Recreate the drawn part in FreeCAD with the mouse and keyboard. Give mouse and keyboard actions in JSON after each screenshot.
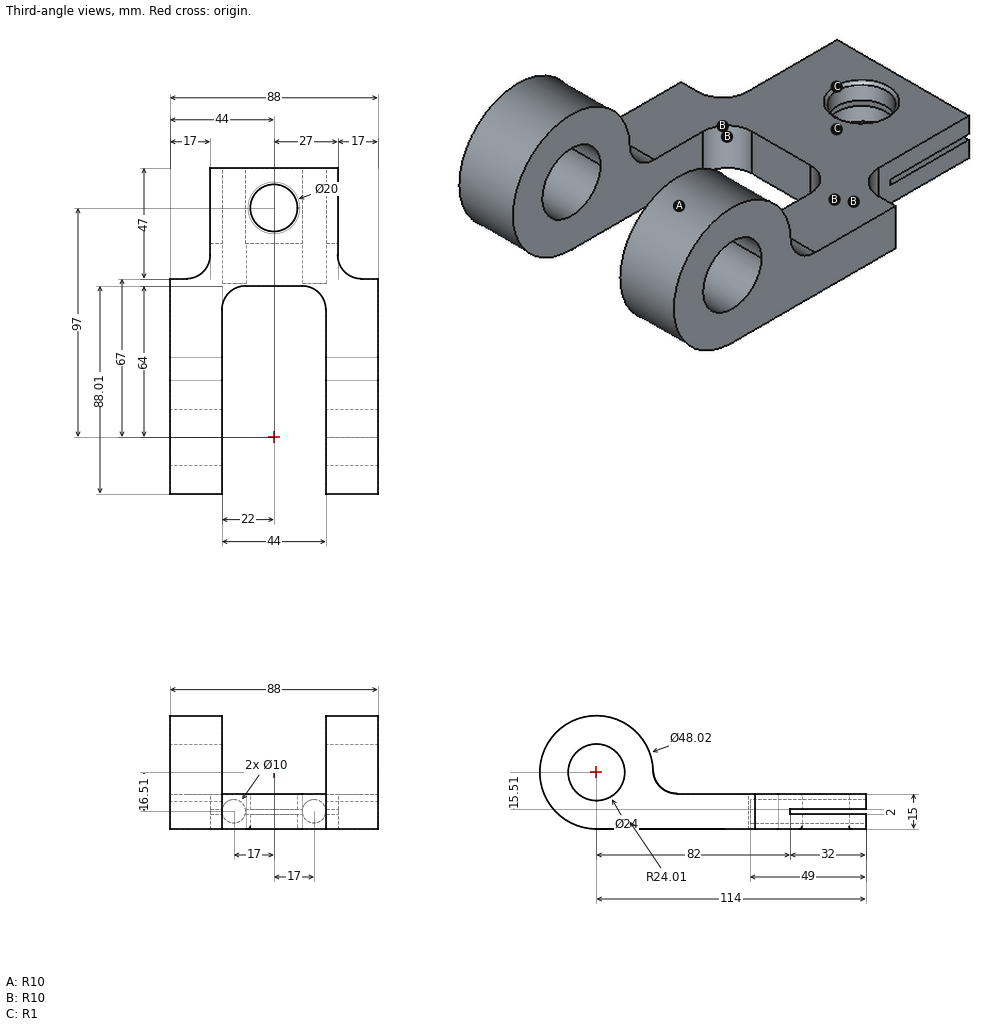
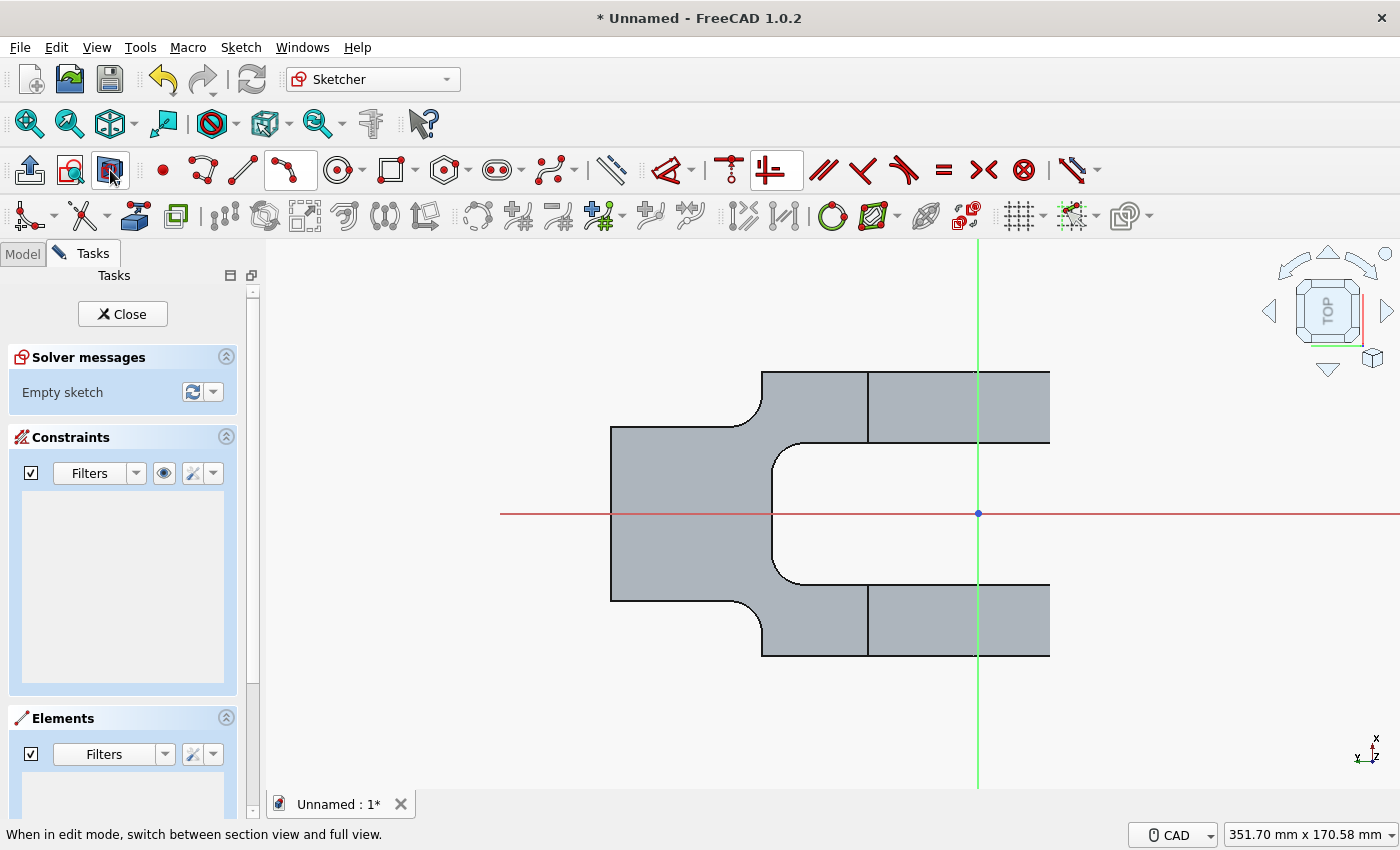
{"action": "scroll", "coordinate": [640, 514], "scroll_direction": "up", "scroll_amount": 8}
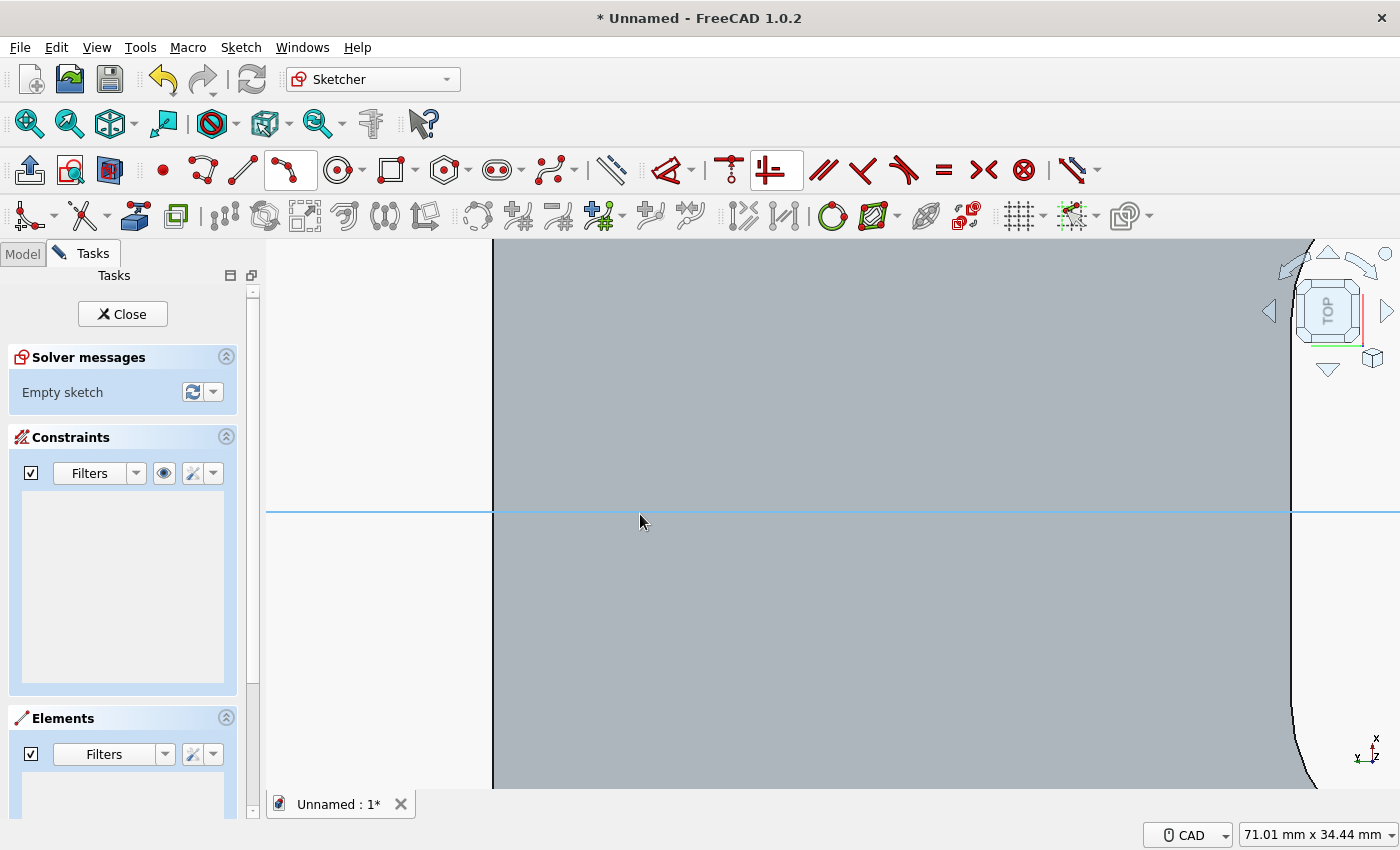
{"action": "left_click", "coordinate": [338, 170]}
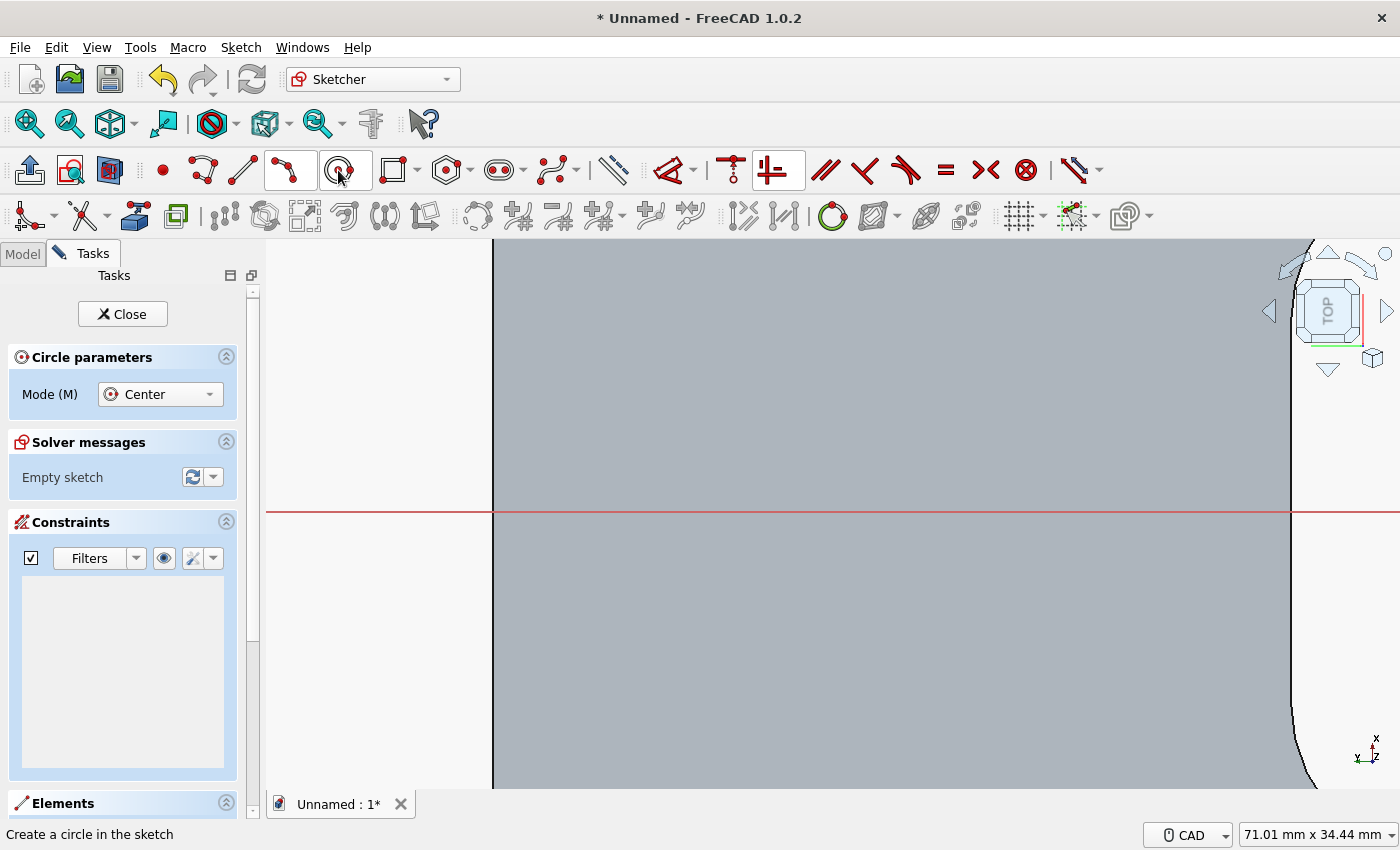
{"action": "left_click", "coordinate": [764, 512]}
{"action": "left_click", "coordinate": [877, 399]}
{"action": "key", "text": "Escape"}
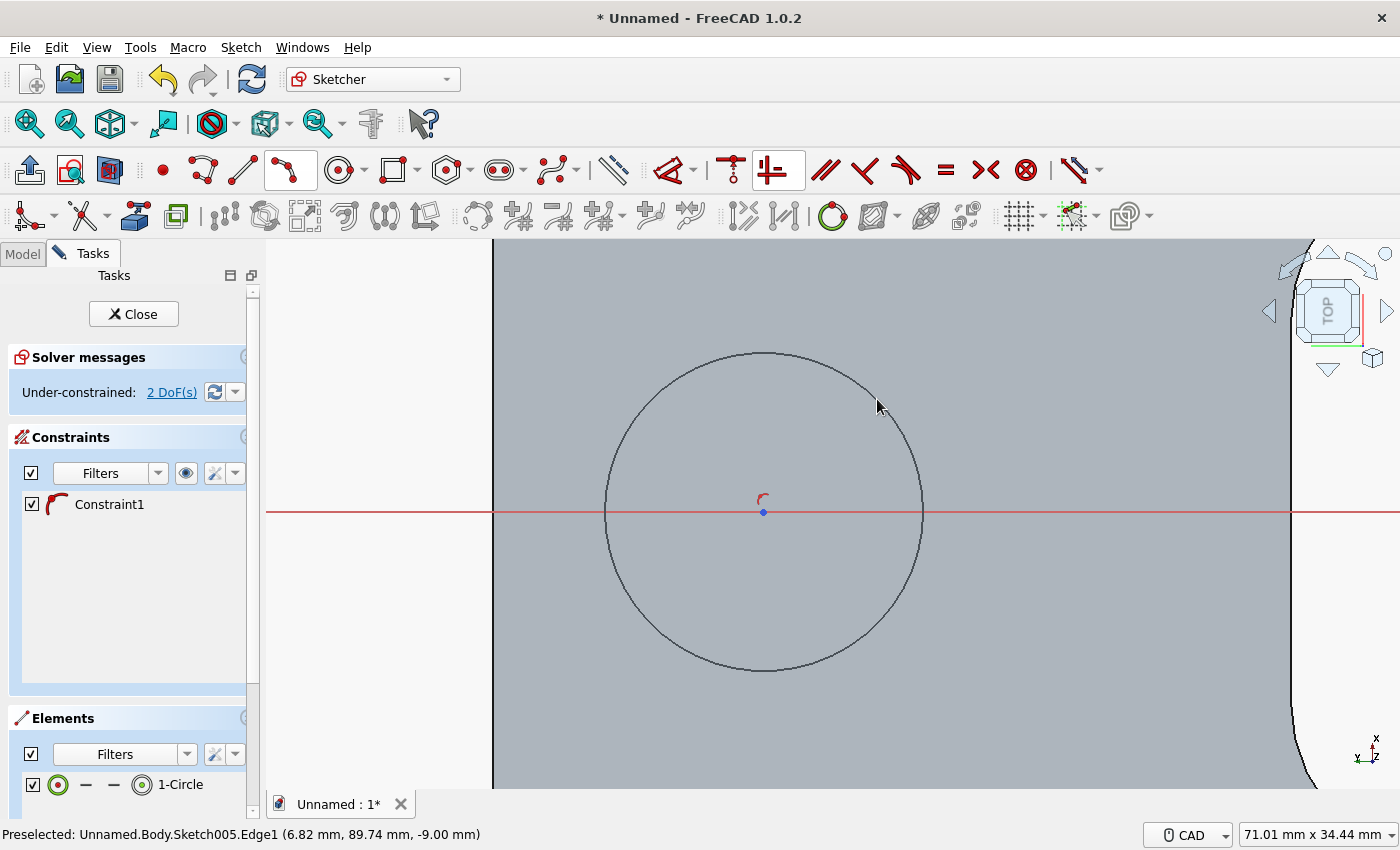
{"action": "left_click", "coordinate": [668, 170]}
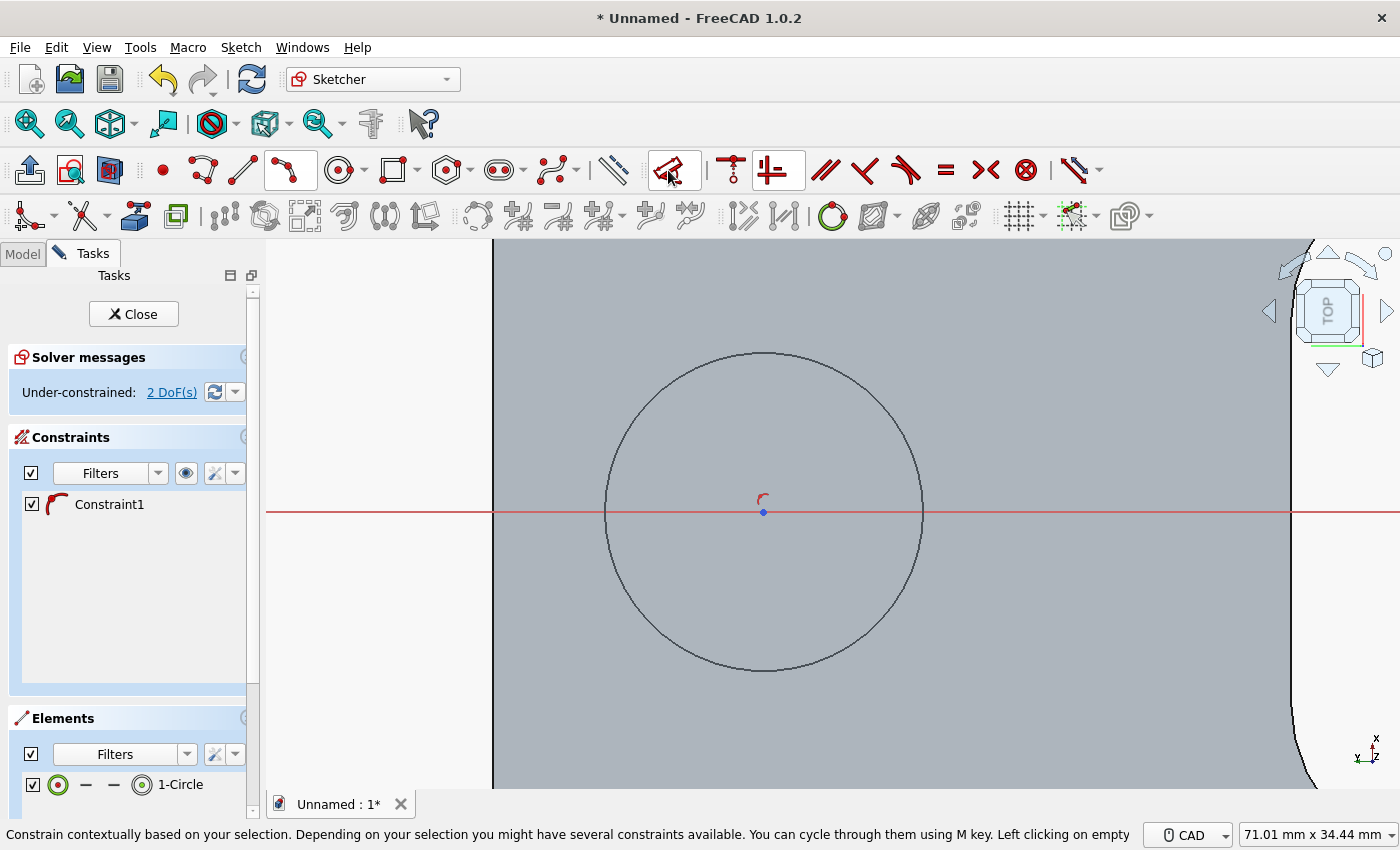
{"action": "left_click", "coordinate": [876, 399]}
{"action": "left_click", "coordinate": [899, 376]}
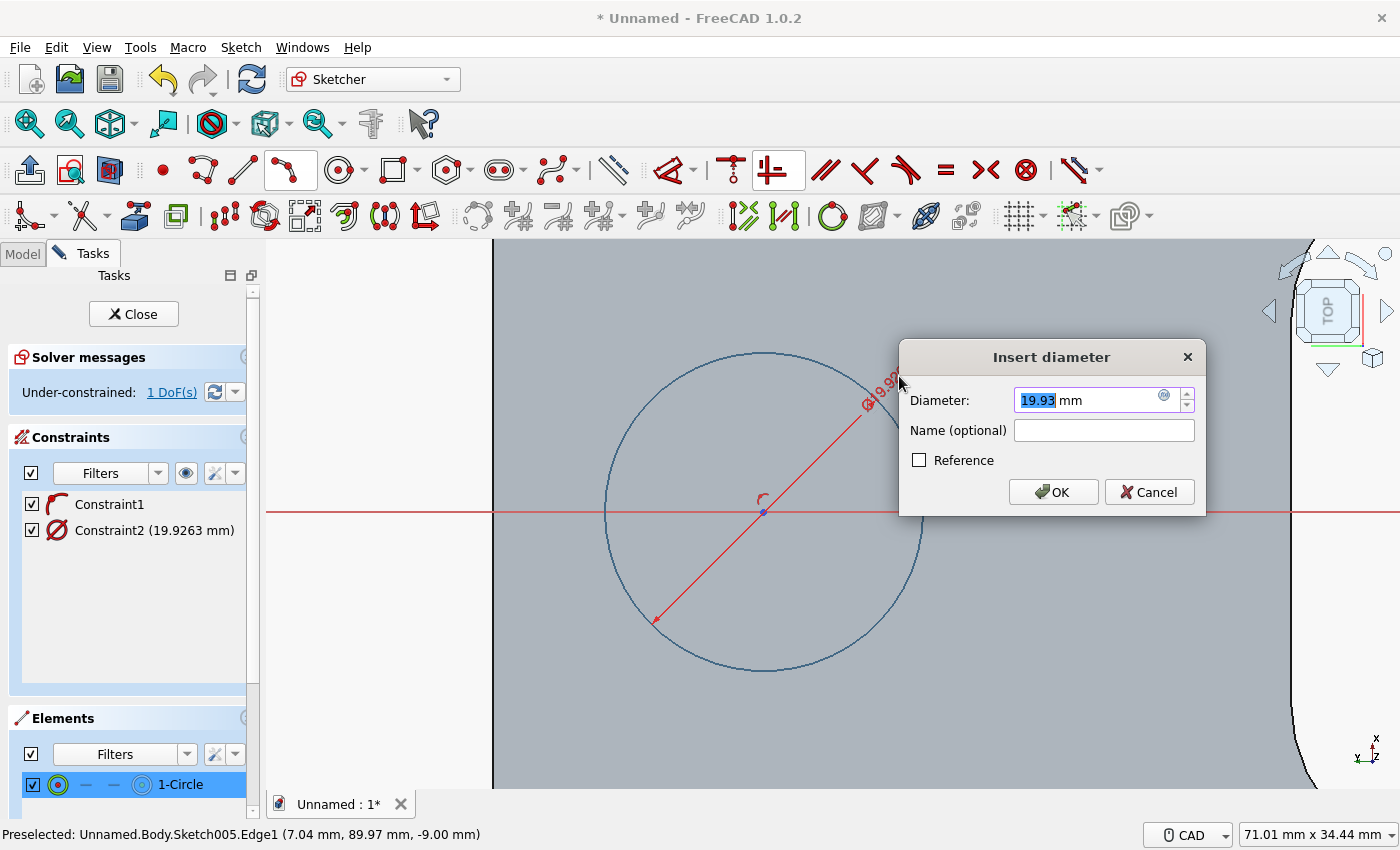
{"action": "type", "text": "20"}
{"action": "key", "text": "Return"}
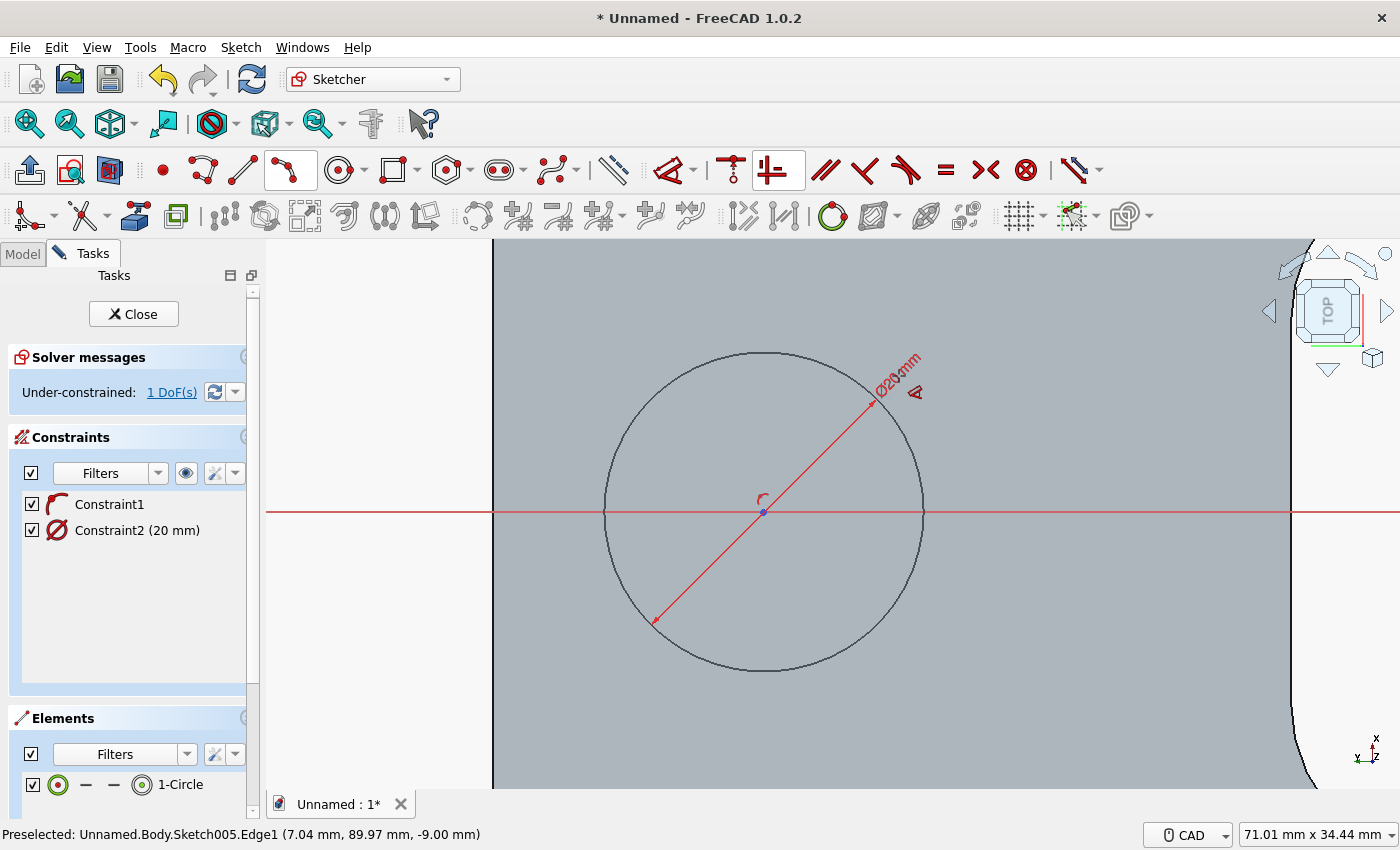
{"action": "left_click", "coordinate": [764, 512]}
{"action": "left_click", "coordinate": [1000, 478]}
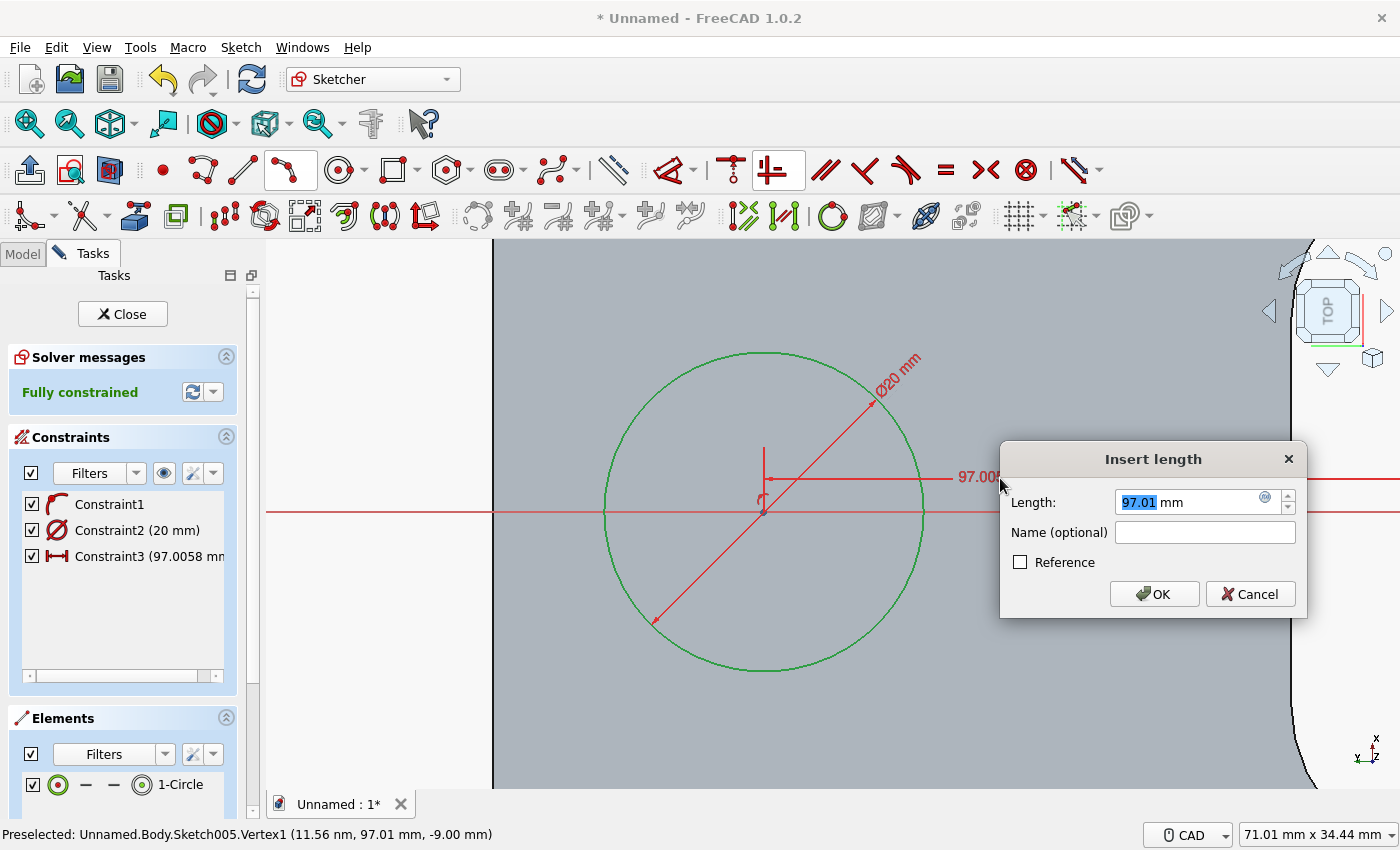
{"action": "type", "text": "97"}
{"action": "key", "text": "Return"}
{"action": "key", "text": "Escape"}